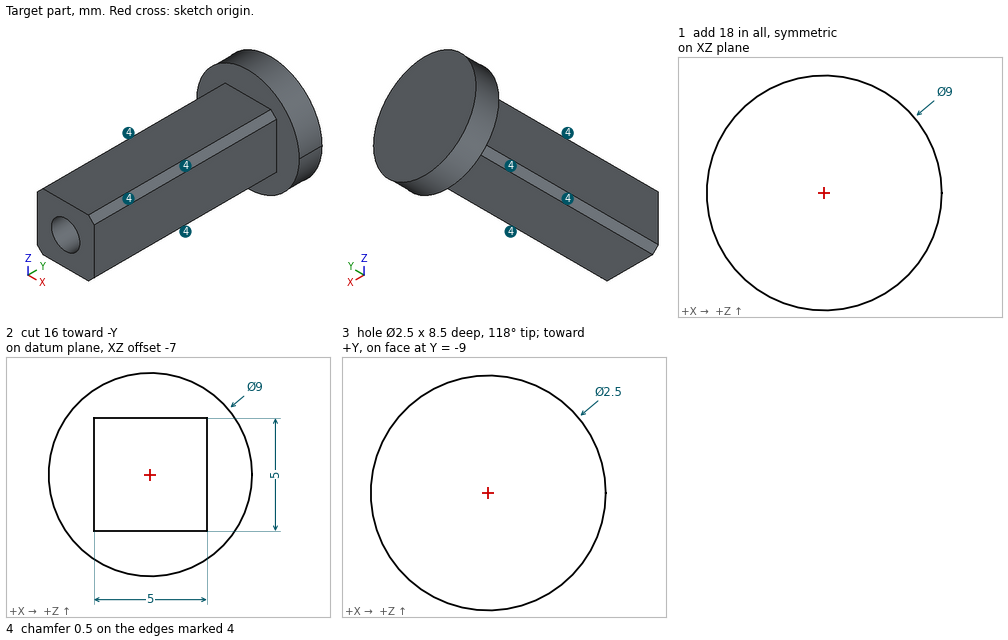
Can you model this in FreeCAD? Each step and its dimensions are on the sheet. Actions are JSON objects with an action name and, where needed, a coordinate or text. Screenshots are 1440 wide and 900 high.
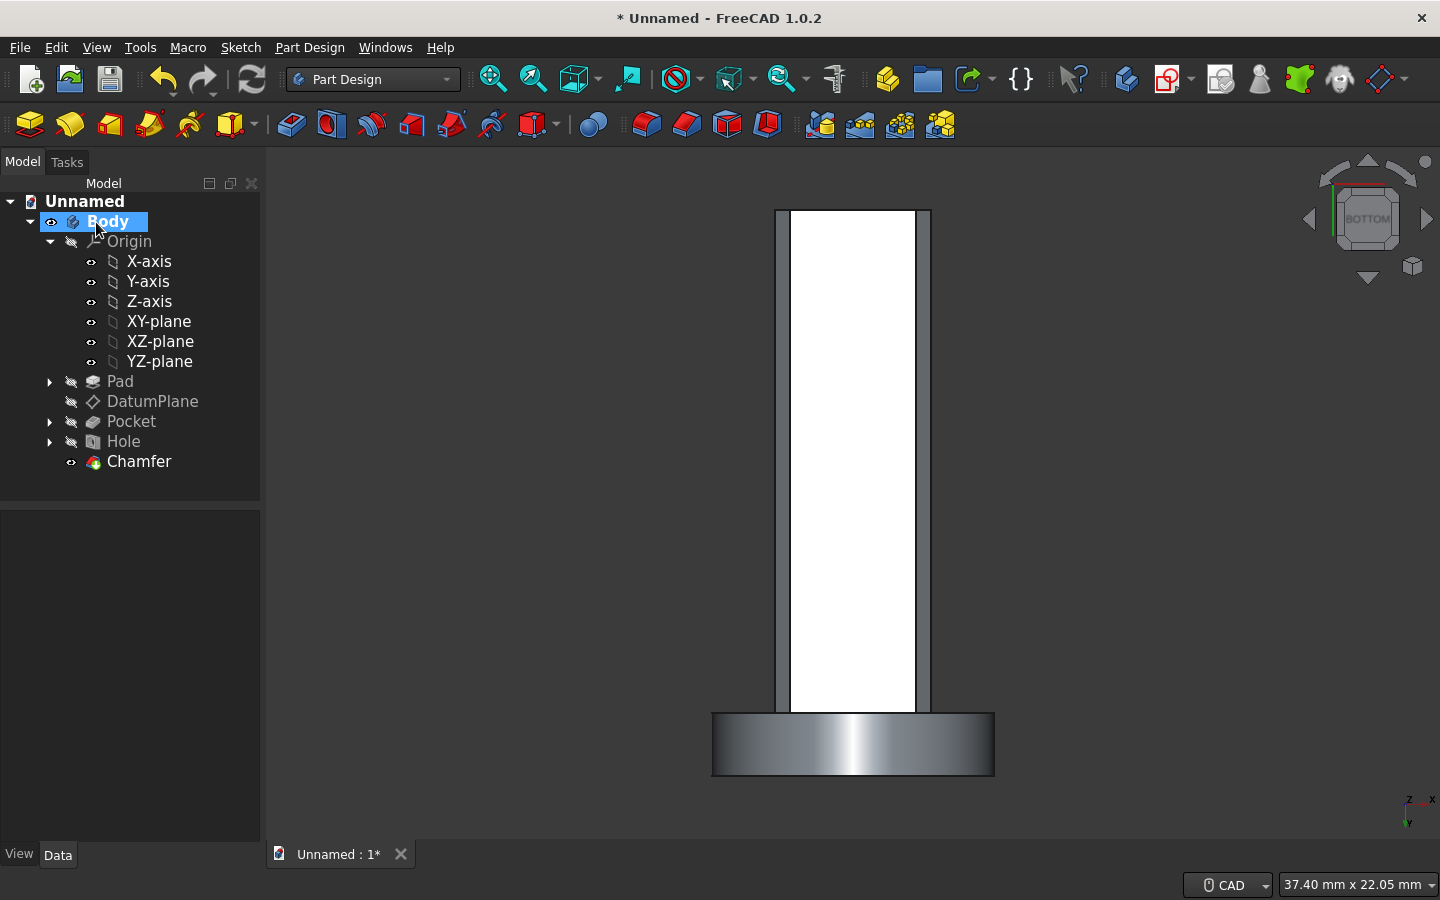
{"action": "key", "text": "0"}